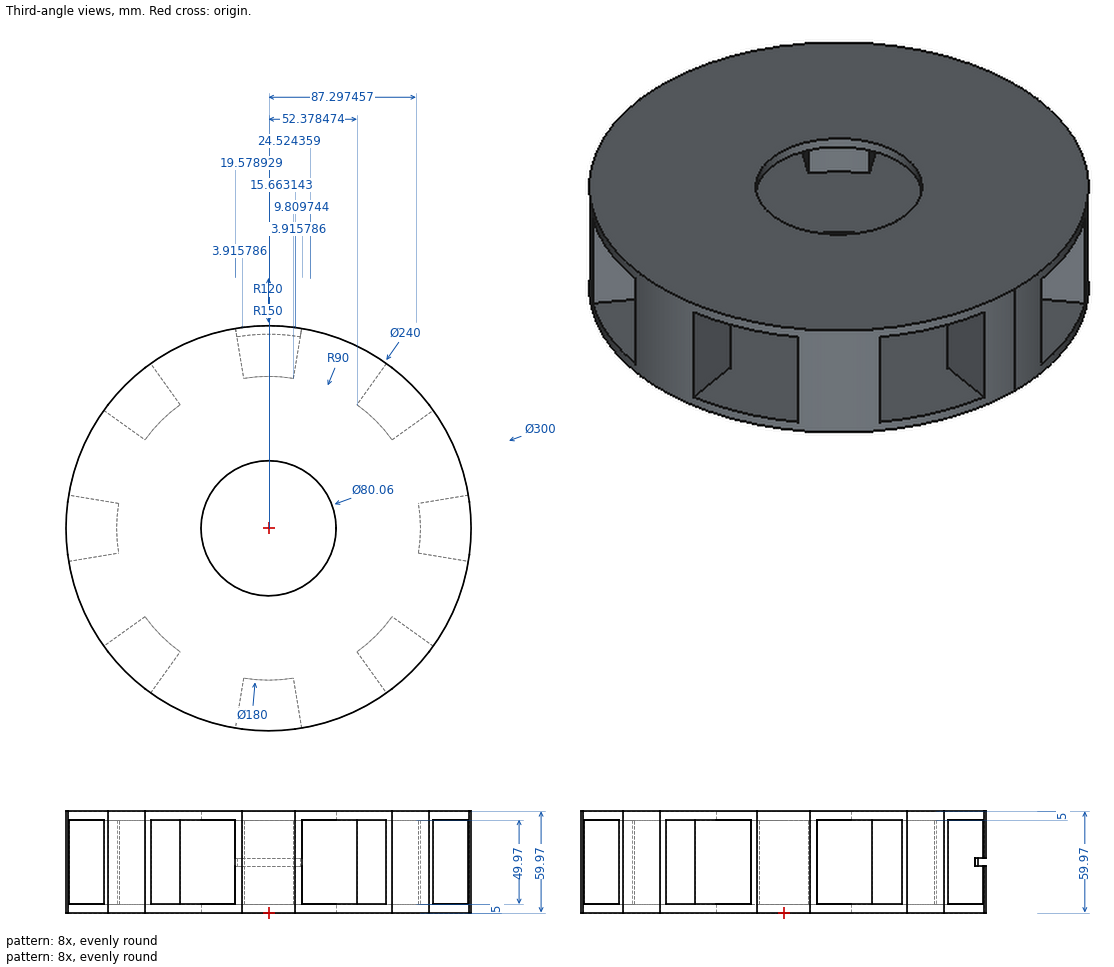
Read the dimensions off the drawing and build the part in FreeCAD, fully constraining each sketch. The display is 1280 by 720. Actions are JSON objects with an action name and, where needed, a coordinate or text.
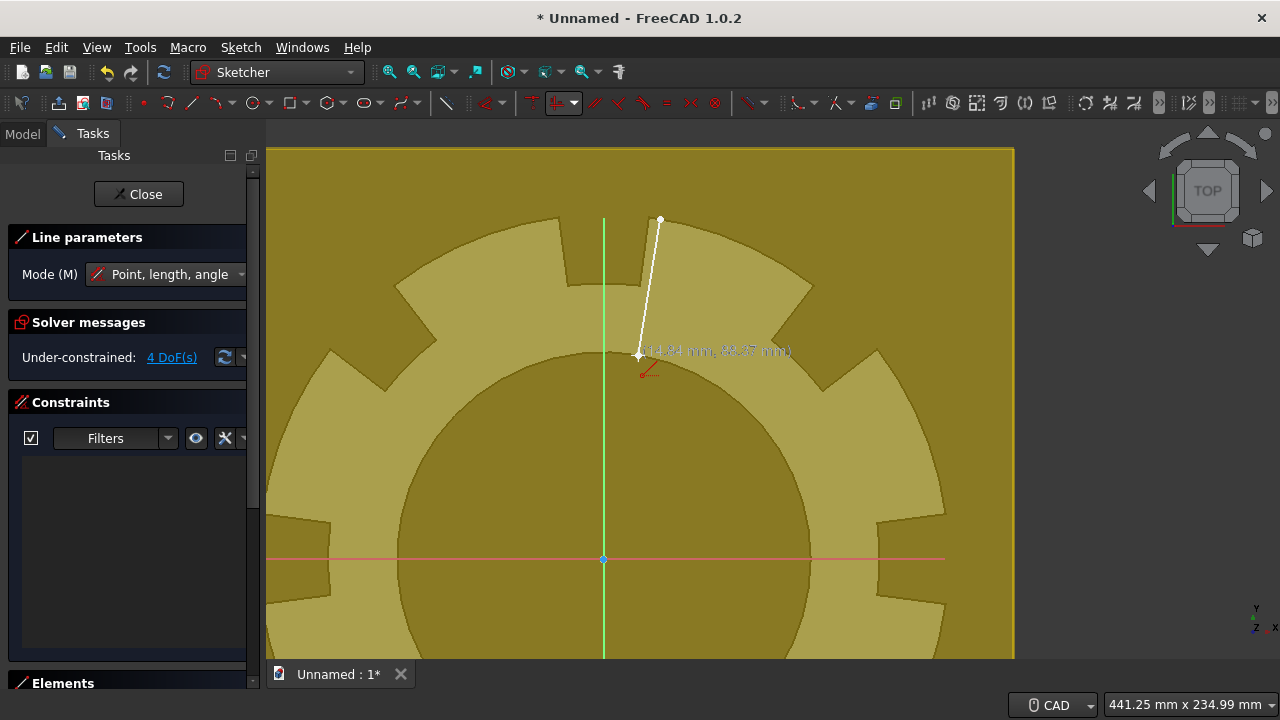
{"action": "left_click", "coordinate": [724, 391]}
{"action": "left_click", "coordinate": [804, 279]}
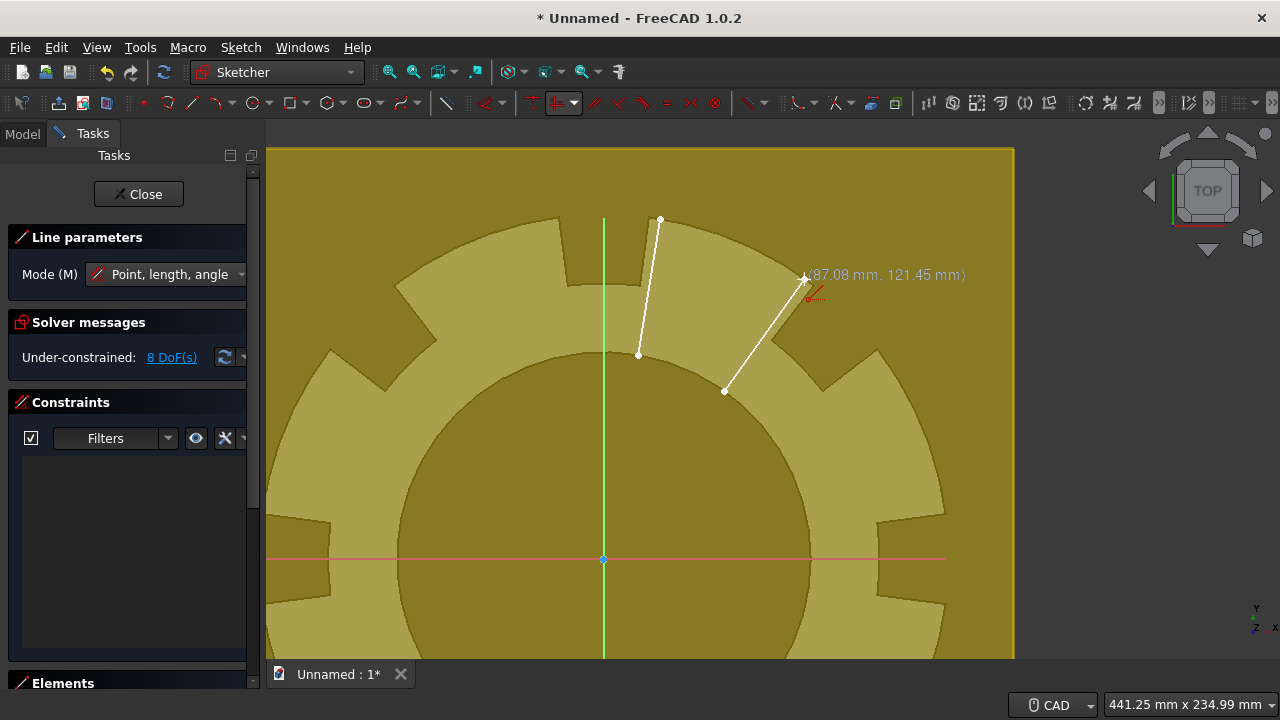
{"action": "left_click", "coordinate": [216, 104]}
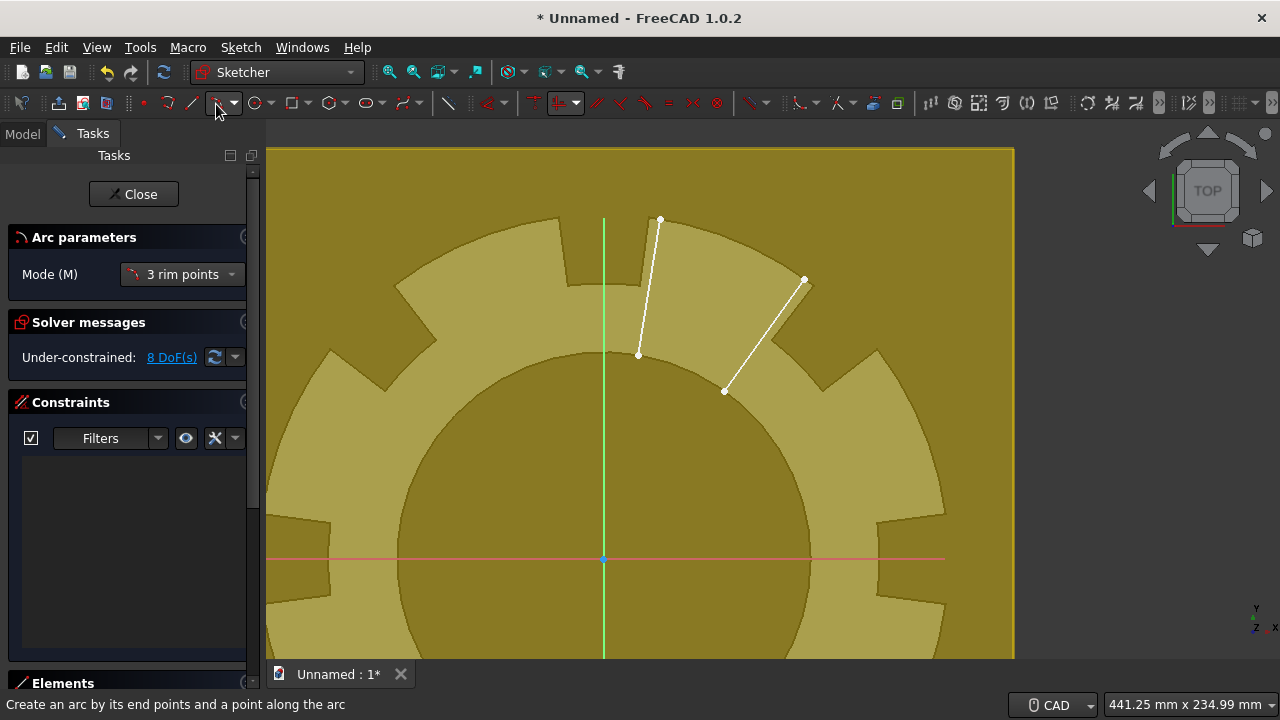
{"action": "left_click", "coordinate": [638, 356]}
{"action": "left_click", "coordinate": [724, 392]}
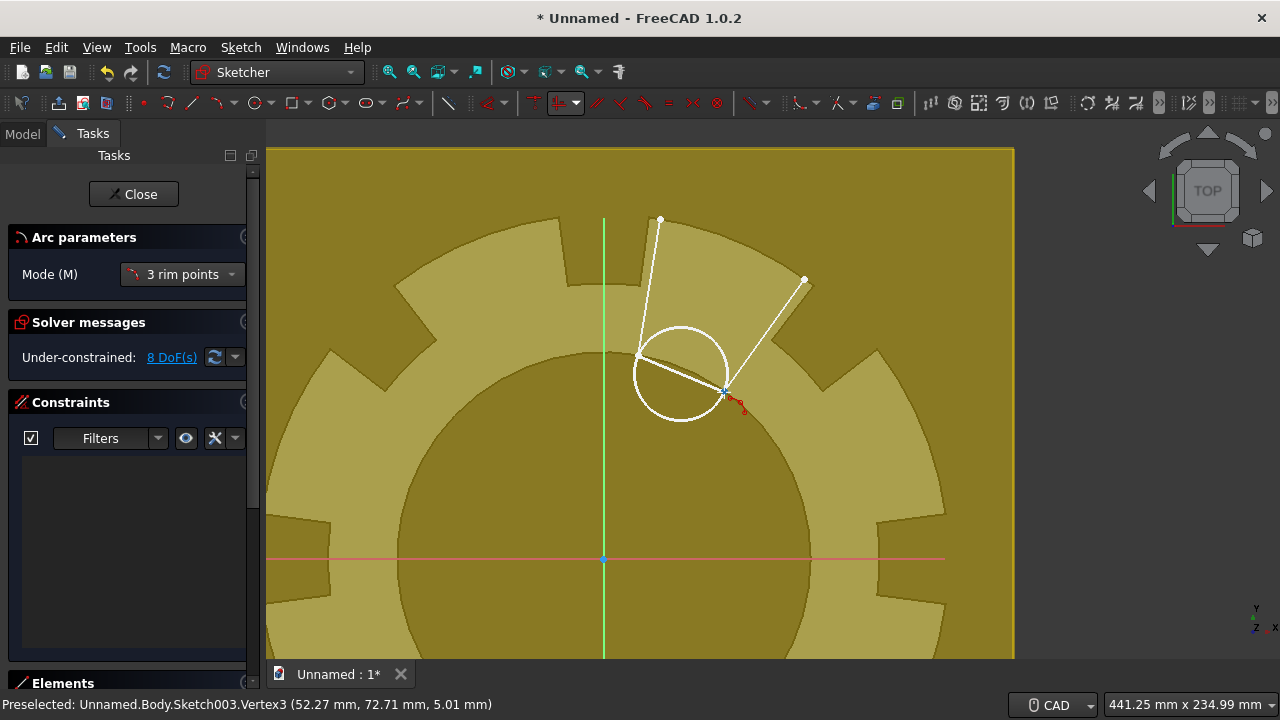
{"action": "scroll", "coordinate": [683, 368], "scroll_direction": "up", "scroll_amount": 6}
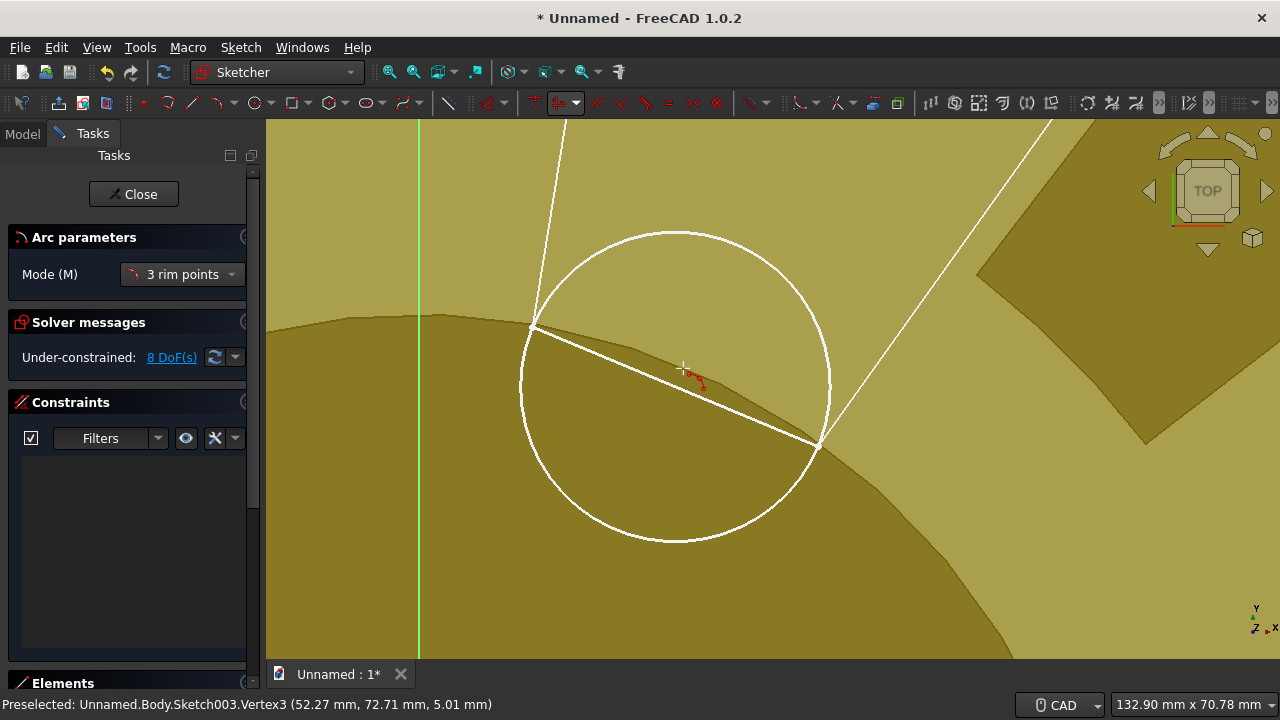
{"action": "left_click", "coordinate": [682, 367]}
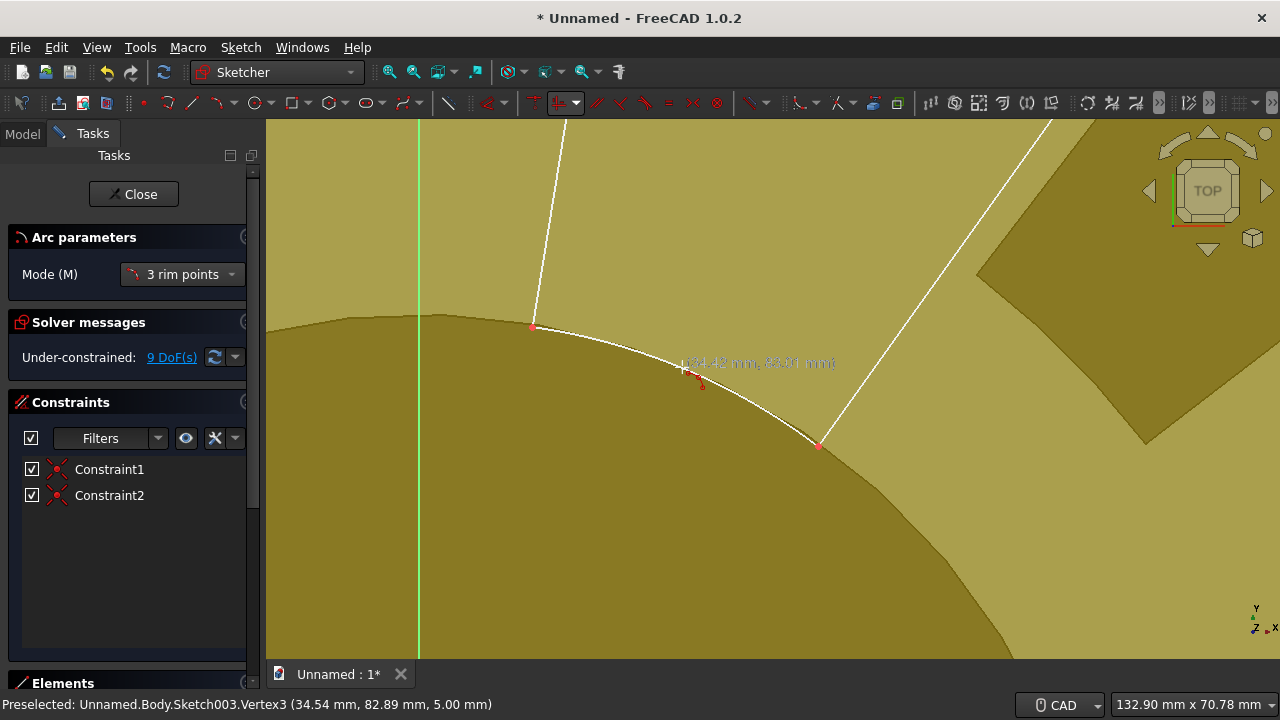
{"action": "scroll", "coordinate": [684, 368], "scroll_direction": "down", "scroll_amount": 6}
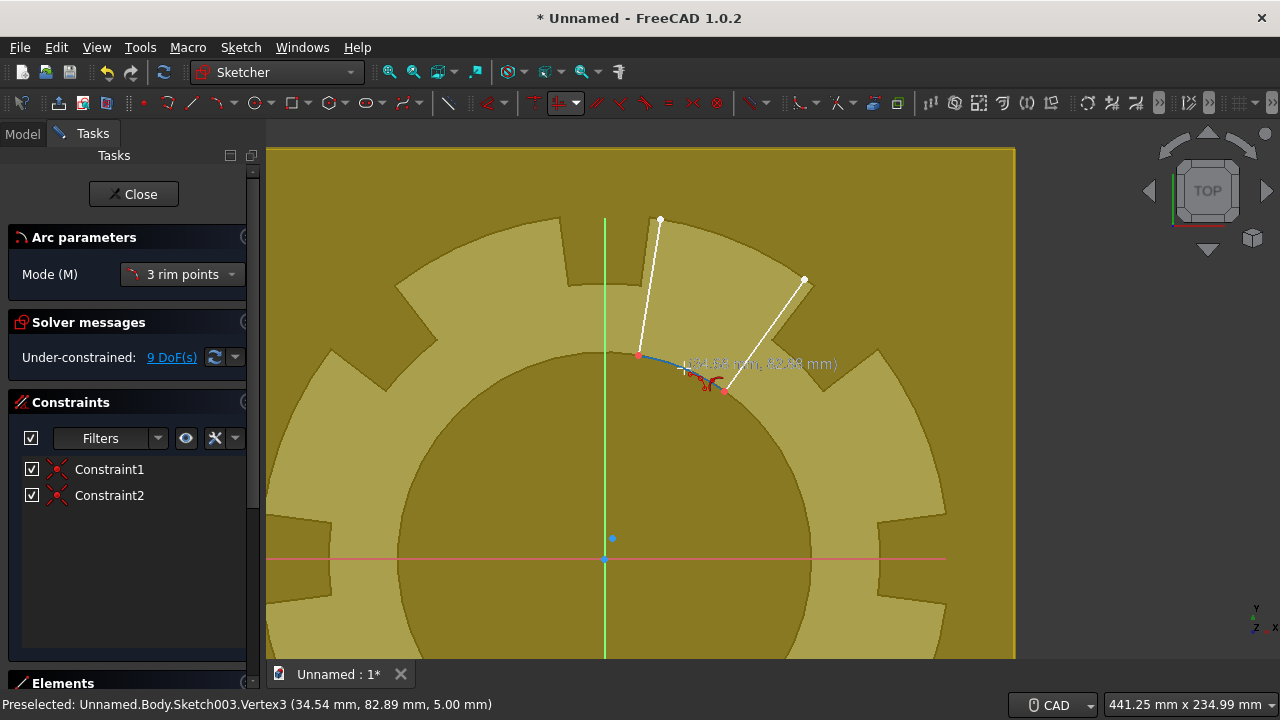
{"action": "left_click", "coordinate": [805, 280]}
{"action": "left_click", "coordinate": [661, 220]}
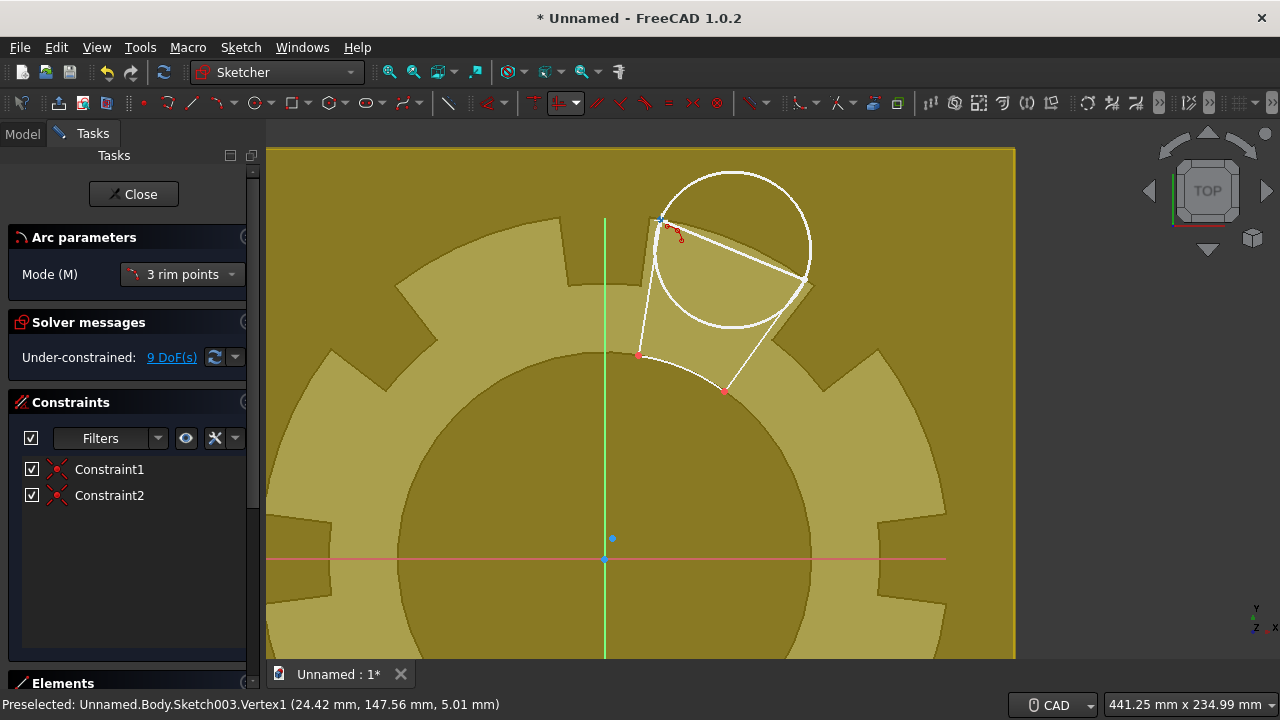
{"action": "scroll", "coordinate": [736, 241], "scroll_direction": "up", "scroll_amount": 3}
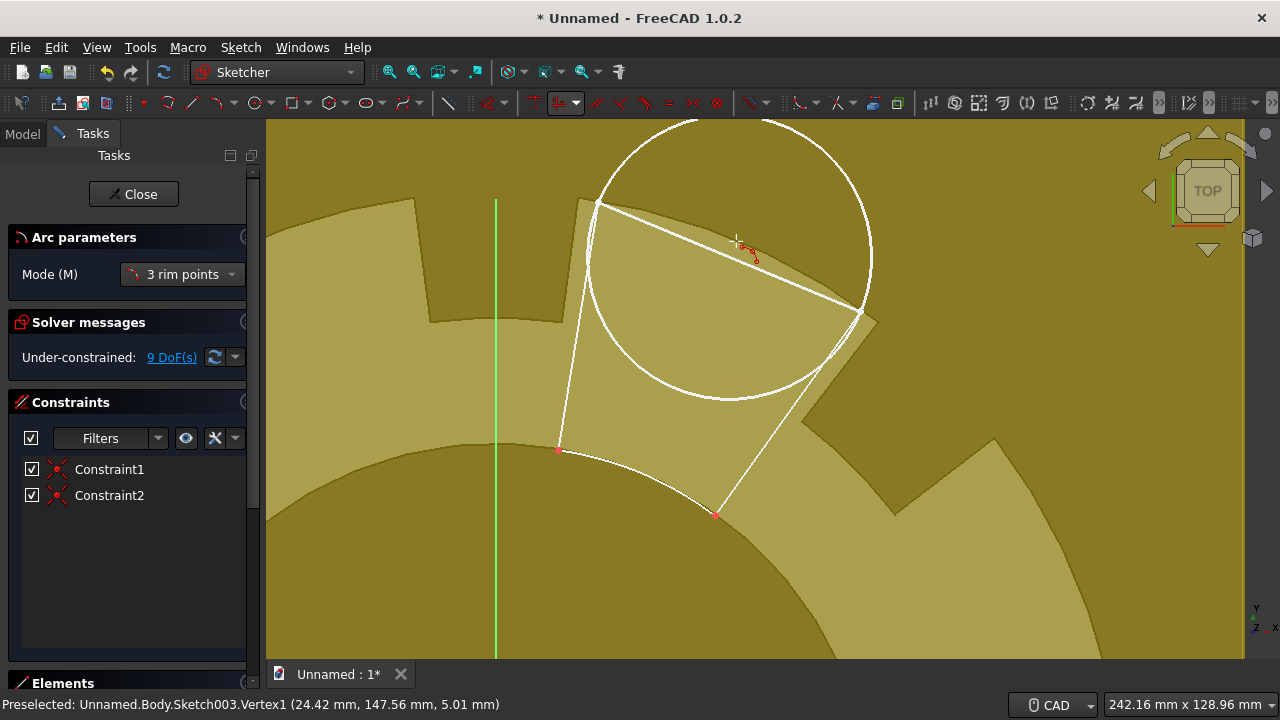
{"action": "left_click", "coordinate": [737, 240]}
{"action": "key", "text": "Escape"}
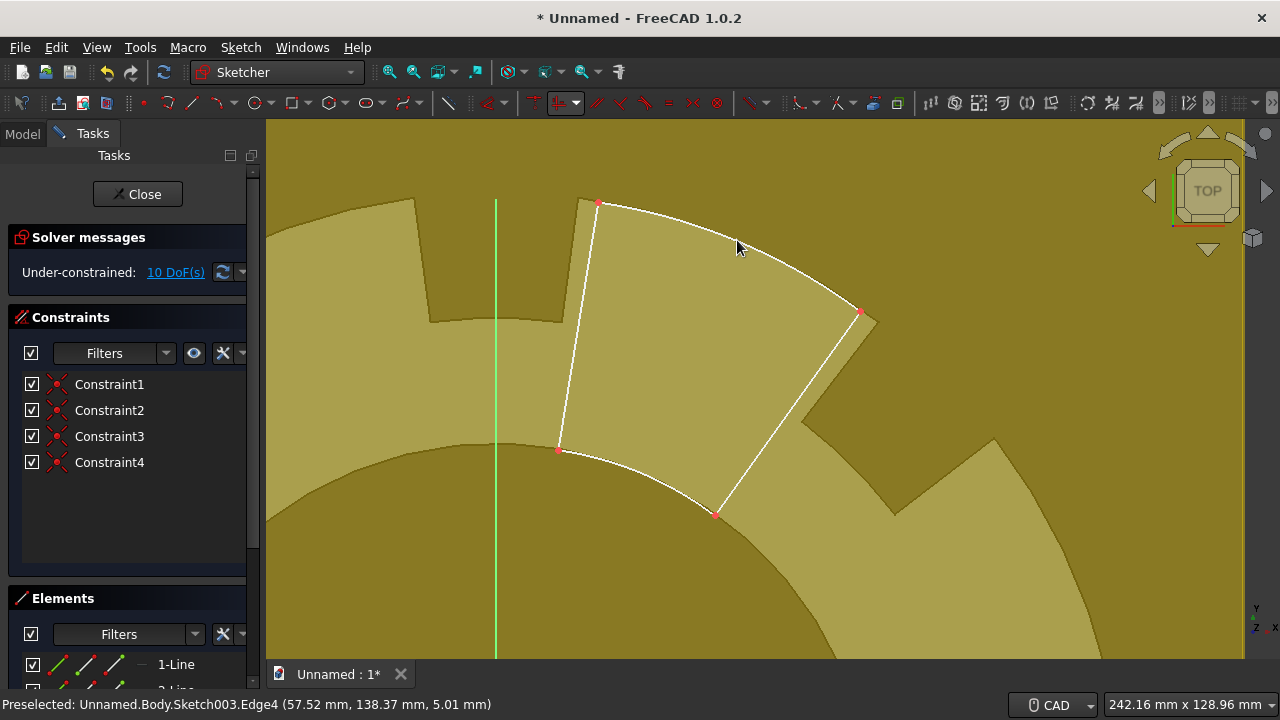
{"action": "left_click", "coordinate": [672, 488]}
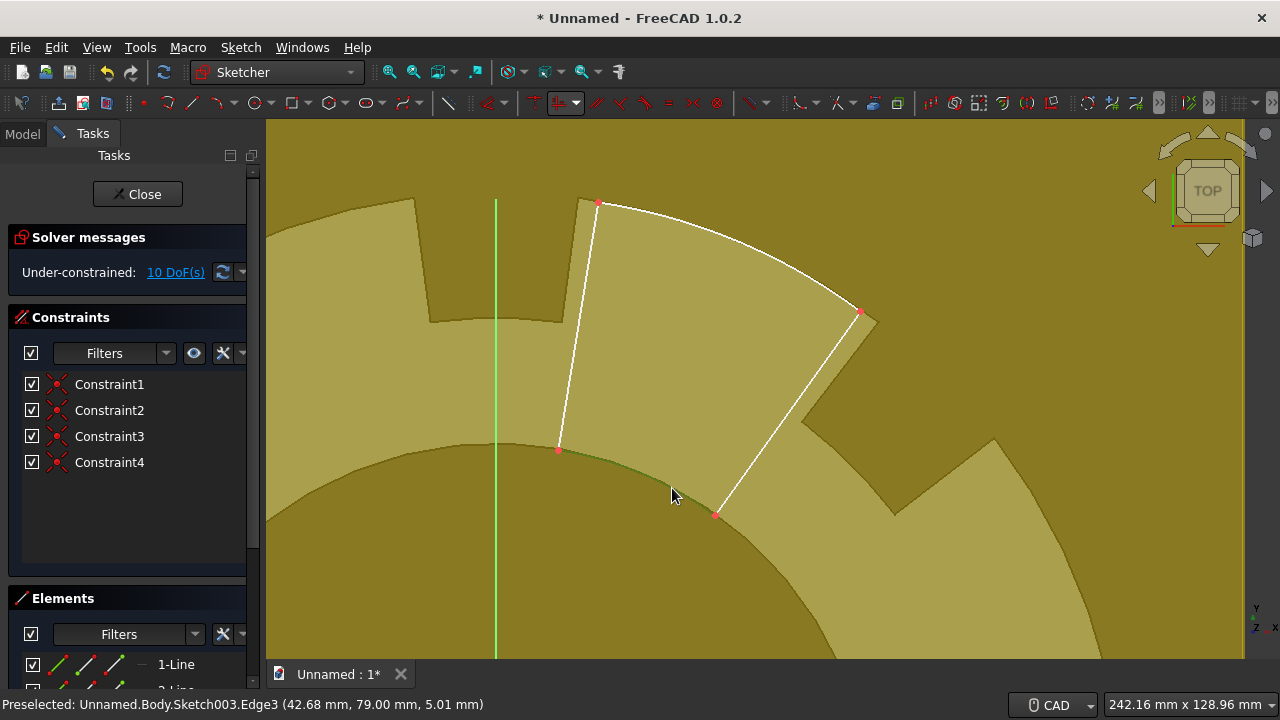
{"action": "left_click", "coordinate": [788, 265]}